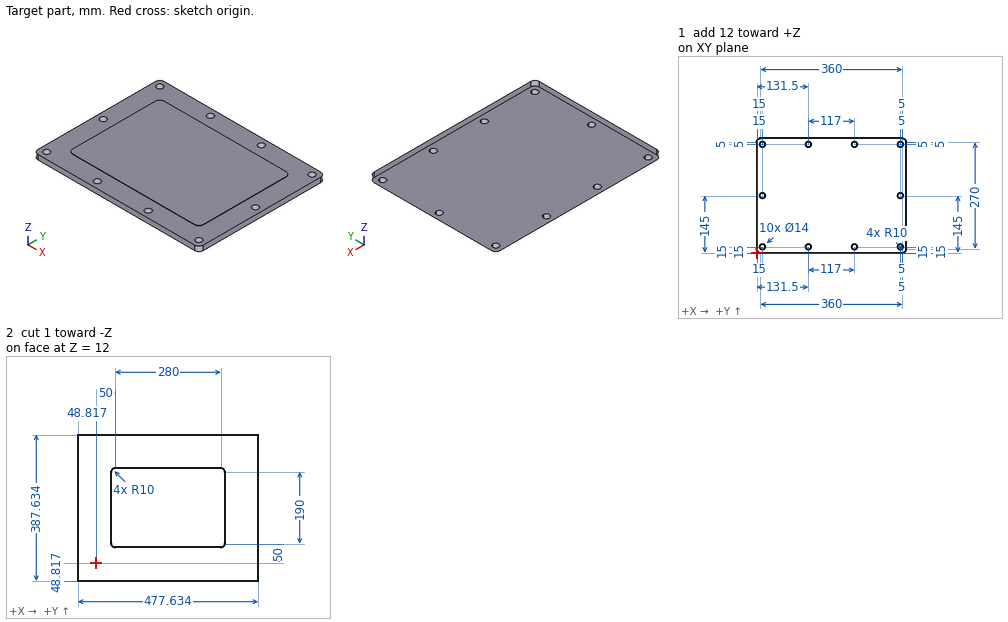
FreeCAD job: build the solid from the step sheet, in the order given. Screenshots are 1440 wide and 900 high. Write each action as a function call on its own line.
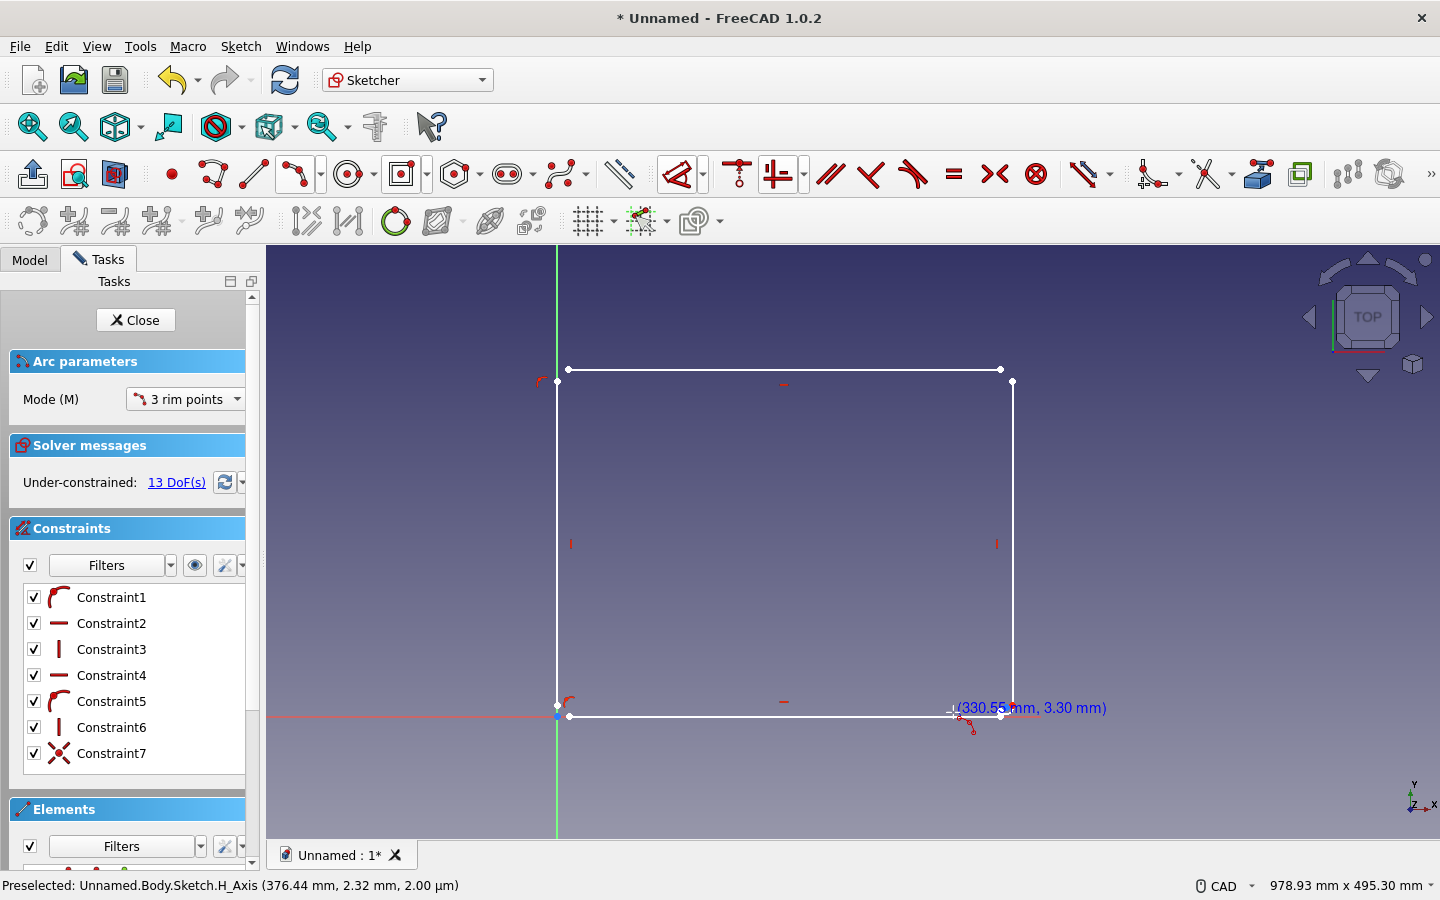
click(1013, 382)
click(1000, 370)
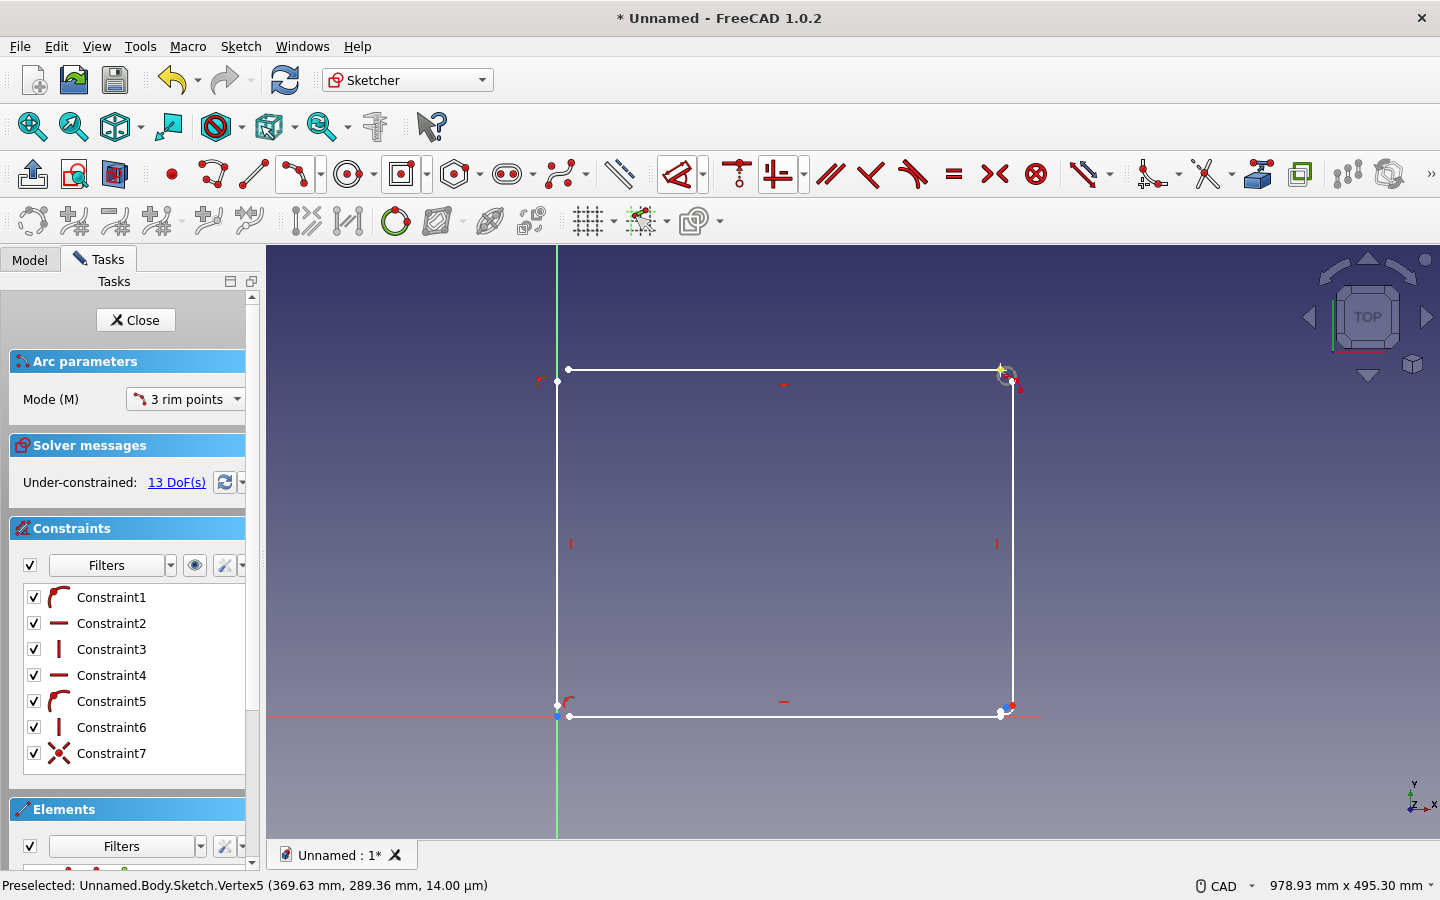
scroll(1009, 373, up, 8)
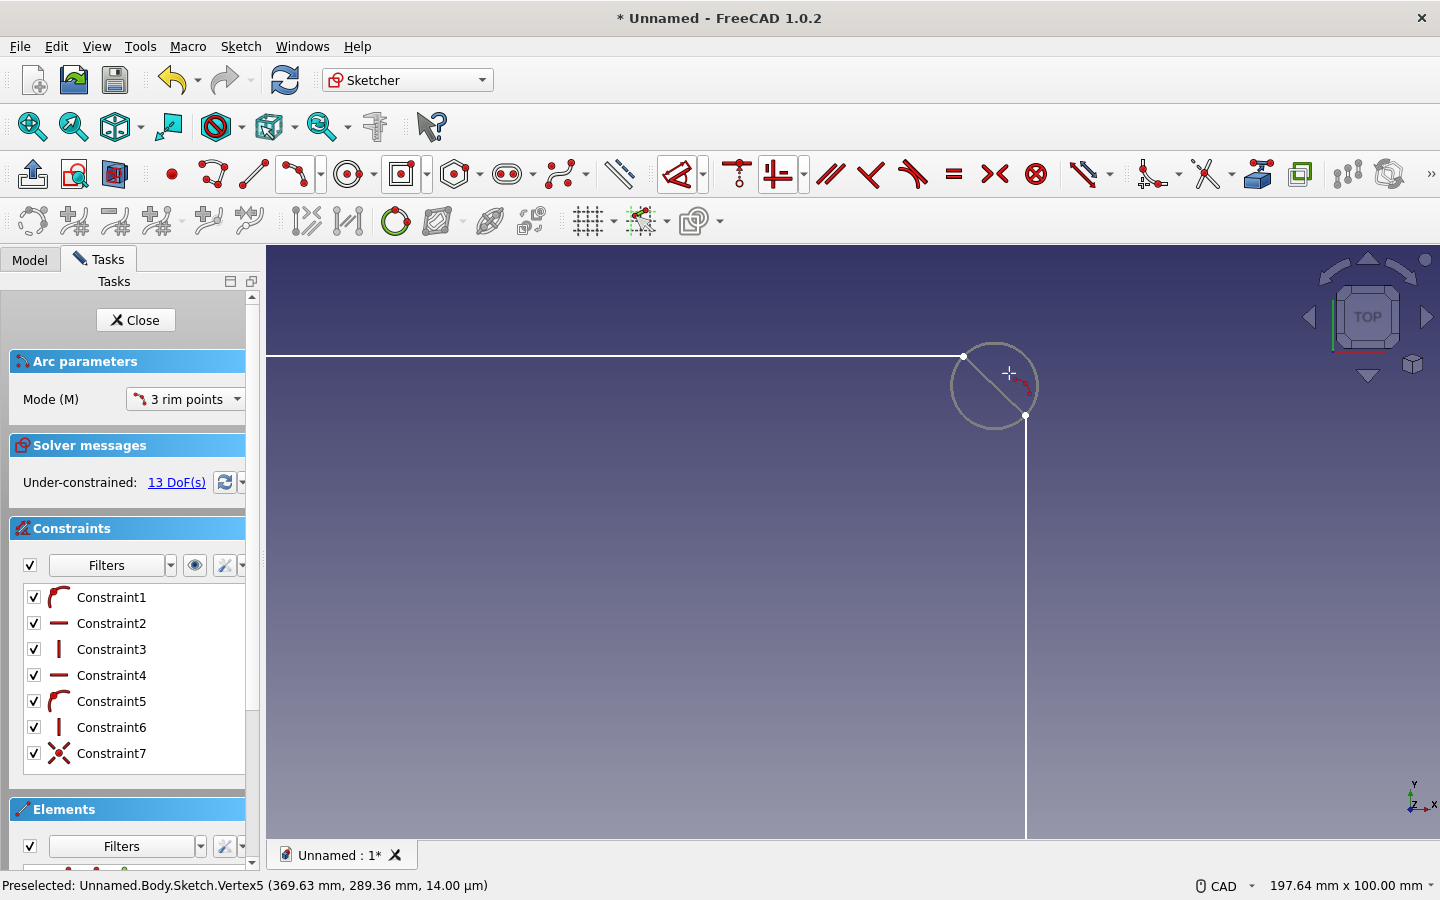
click(1008, 370)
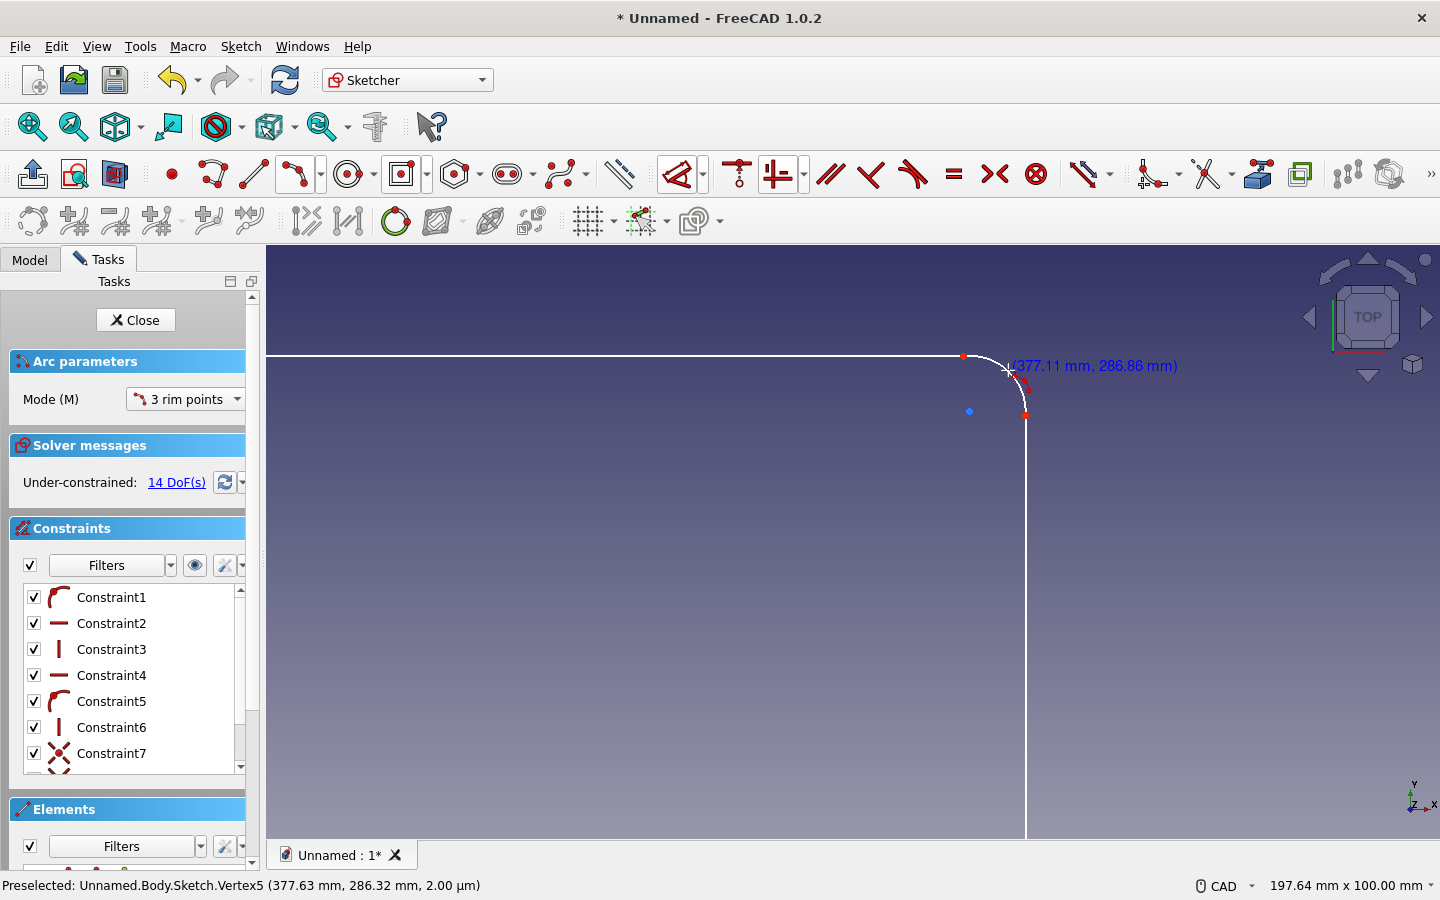
scroll(1009, 372, down, 8)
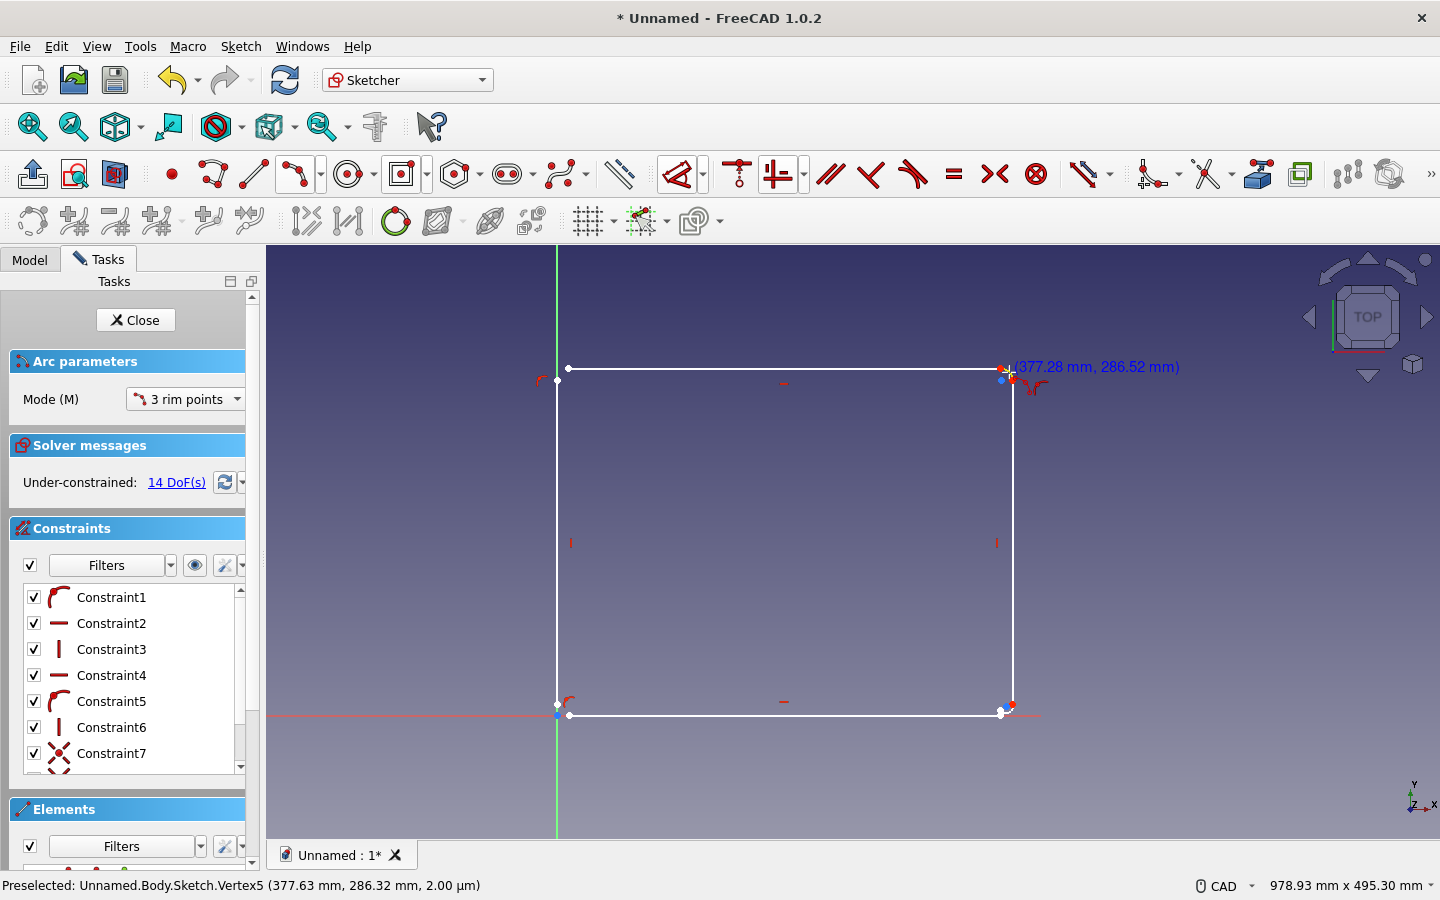
scroll(569, 368, up, 2)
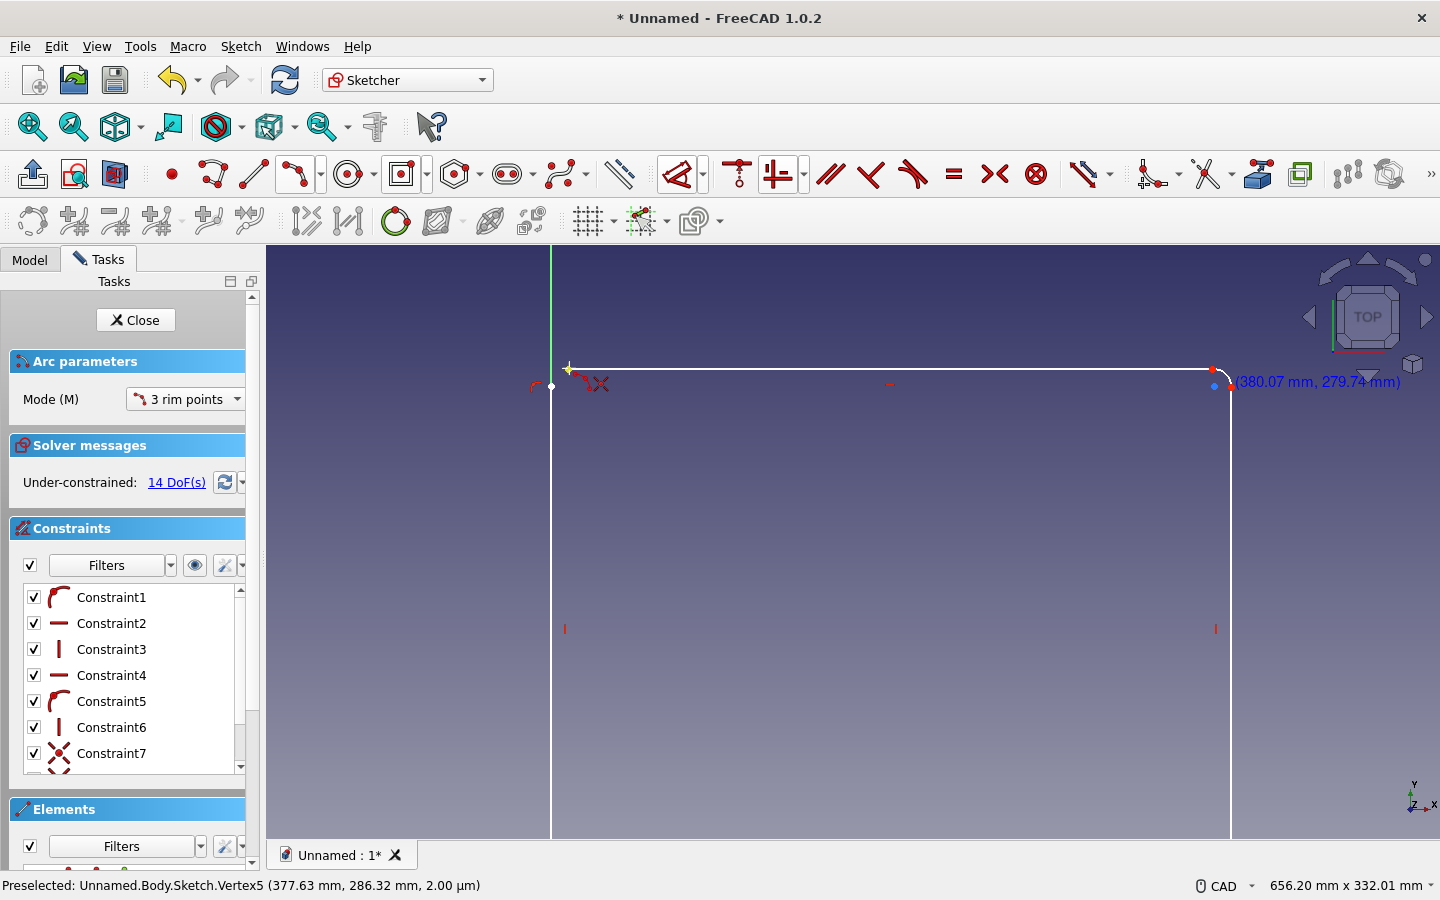
click(568, 369)
click(551, 387)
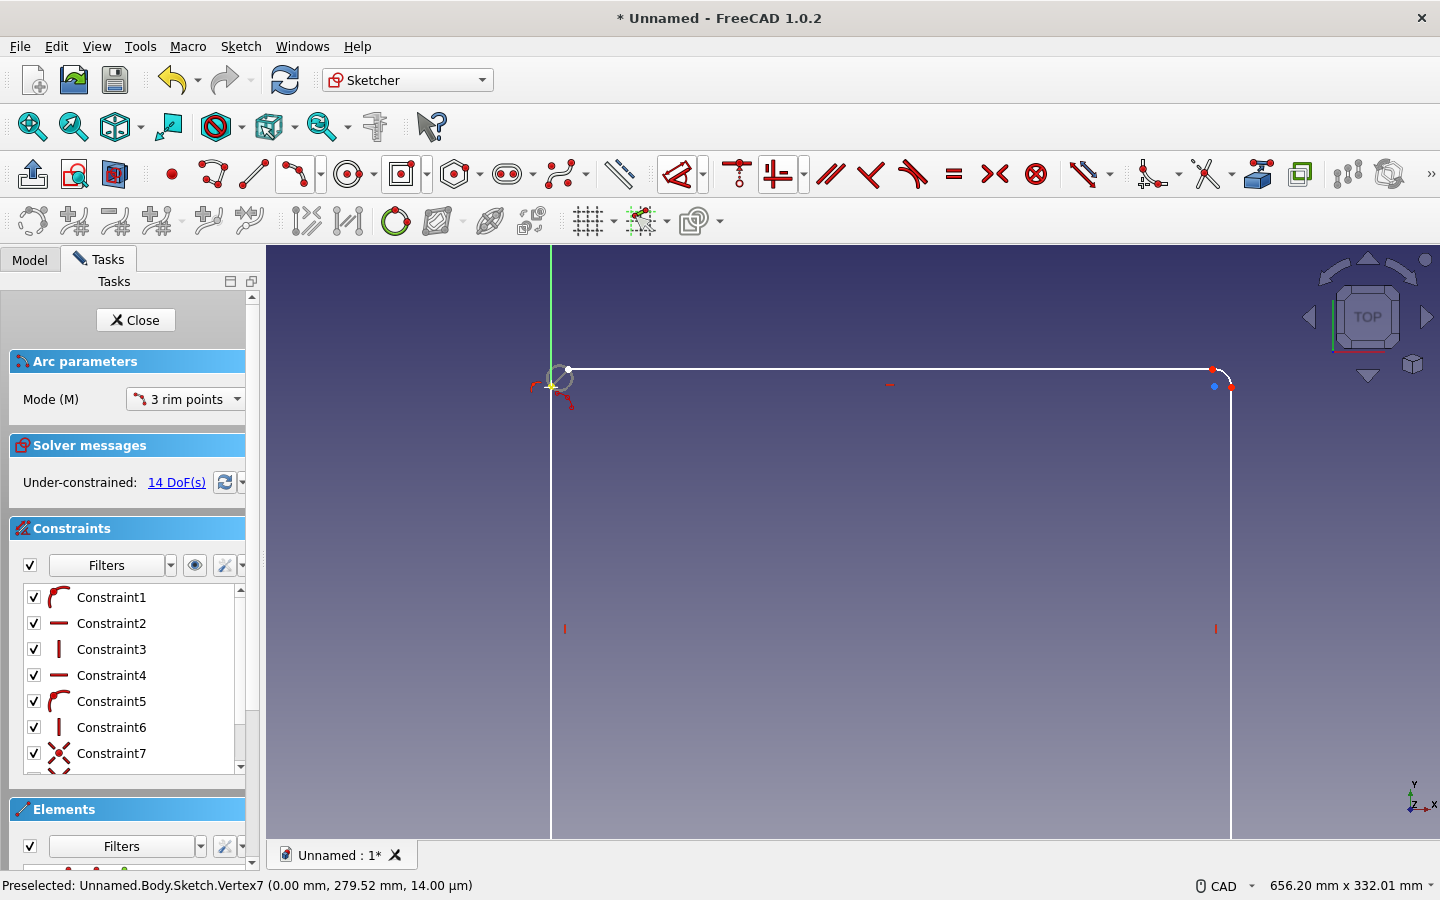
scroll(556, 373, up, 6)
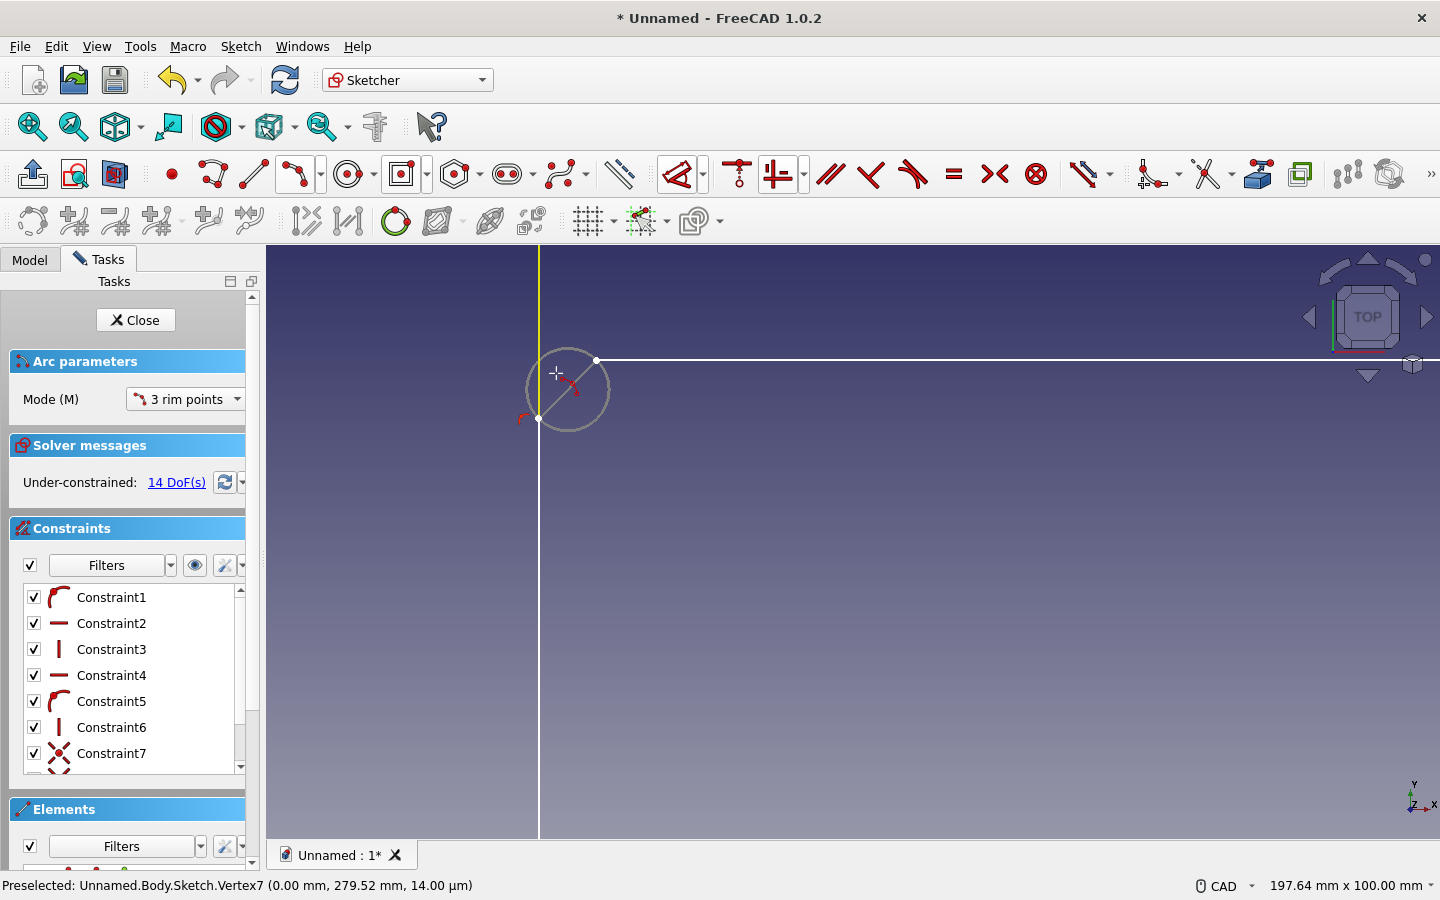
click(556, 374)